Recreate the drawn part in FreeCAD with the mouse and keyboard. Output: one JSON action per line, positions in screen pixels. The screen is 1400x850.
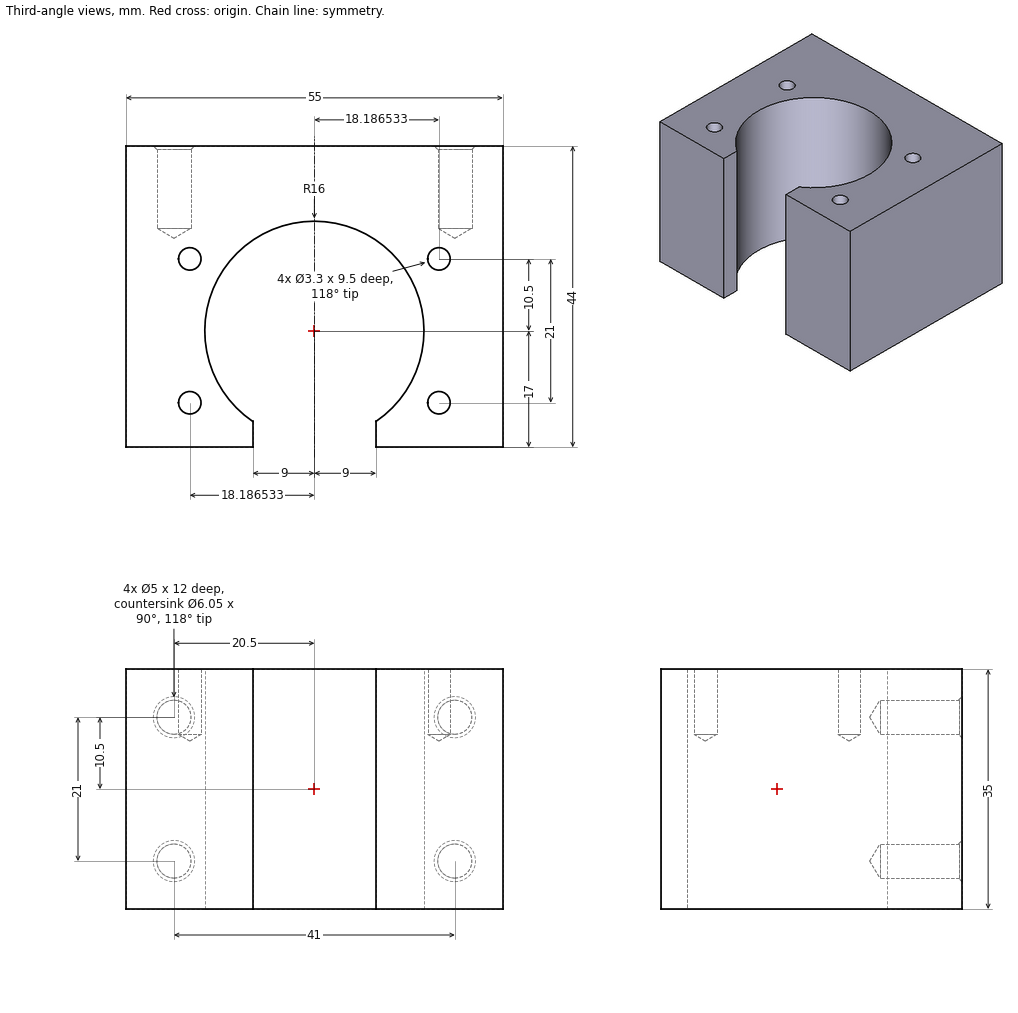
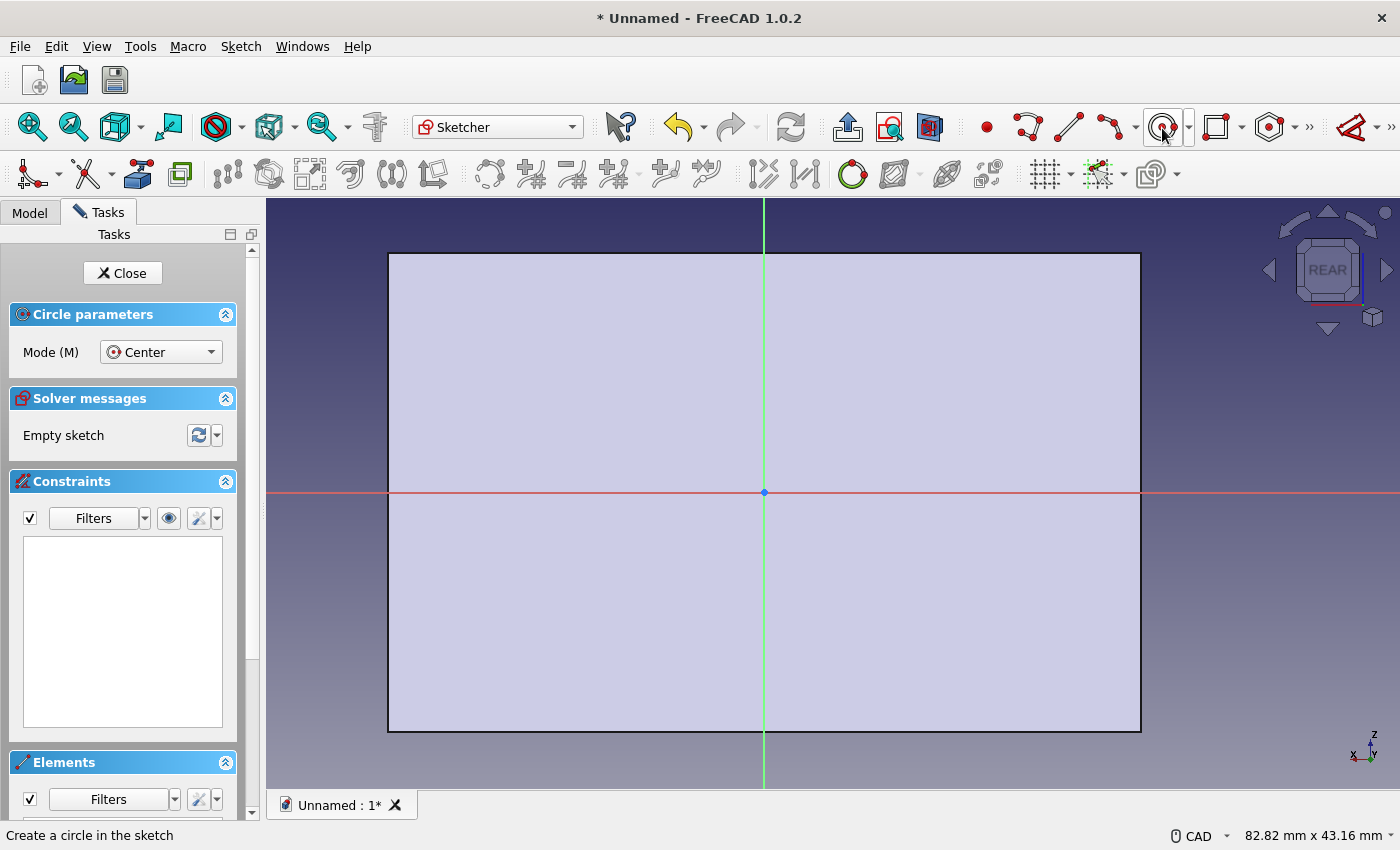
{"action": "left_click", "coordinate": [1045, 349]}
{"action": "mouse_move", "coordinate": [1069, 325]}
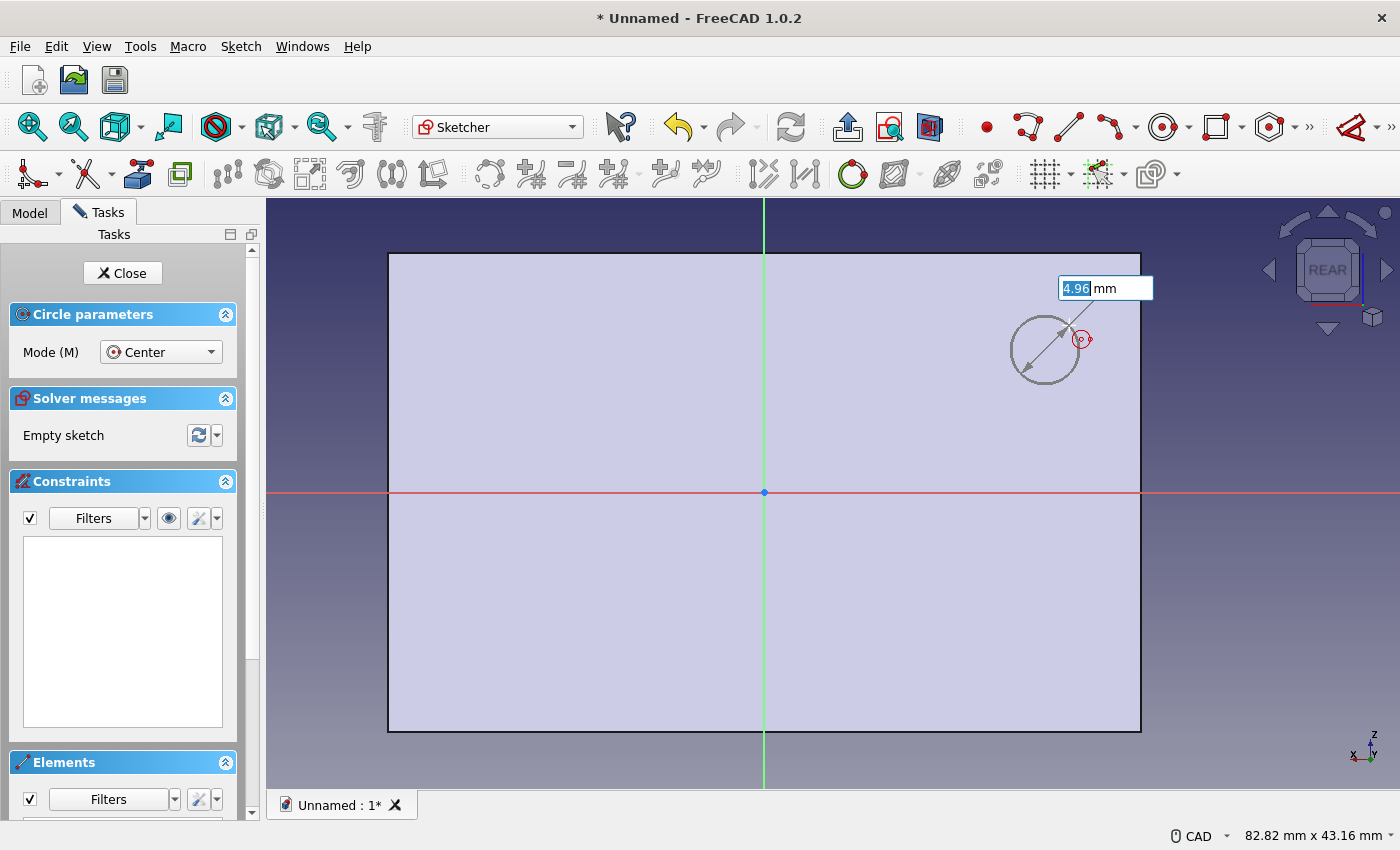
{"action": "type", "text": "5"}
{"action": "key", "text": "Return"}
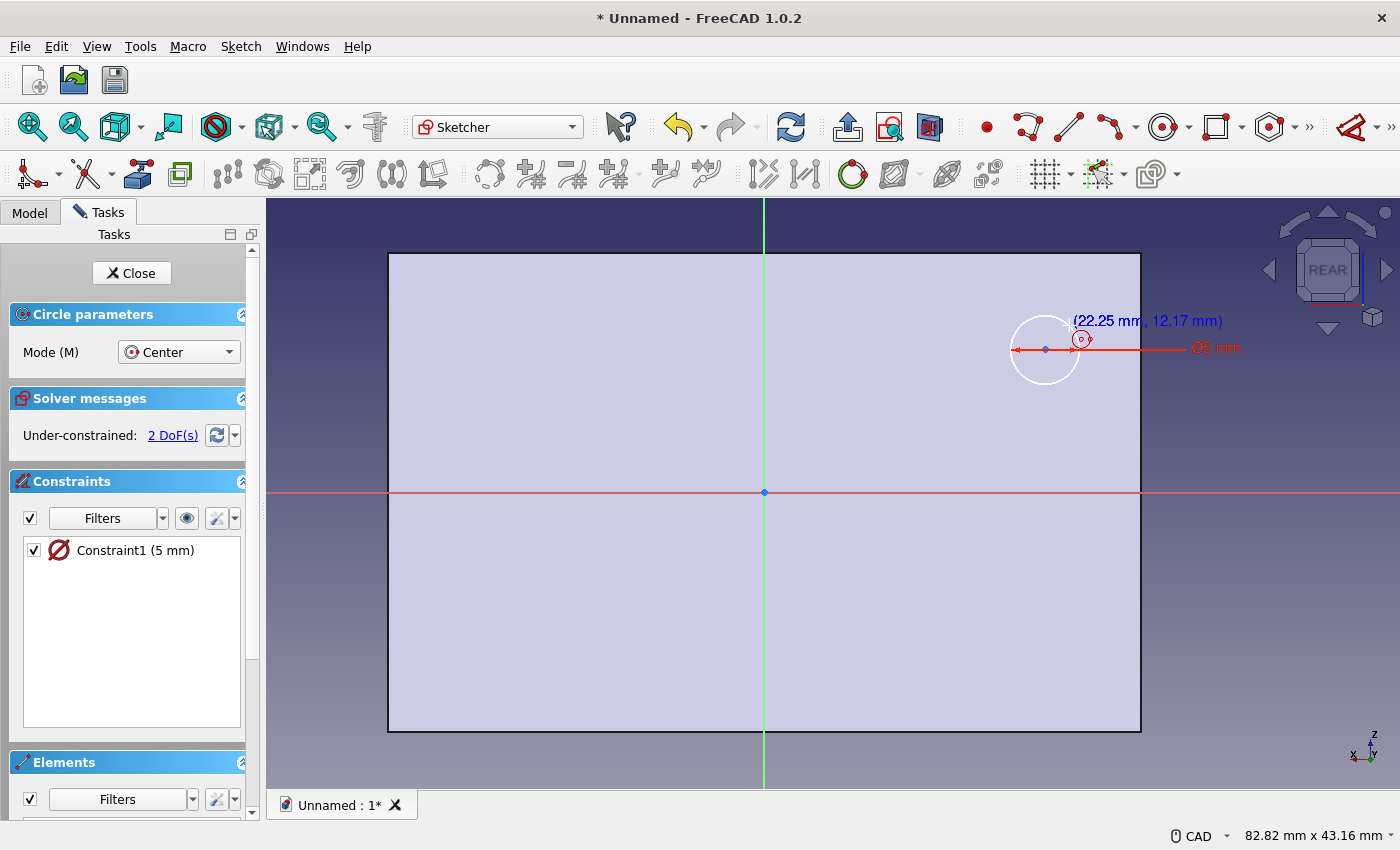
{"action": "left_click", "coordinate": [1045, 636]}
{"action": "mouse_move", "coordinate": [1069, 612]}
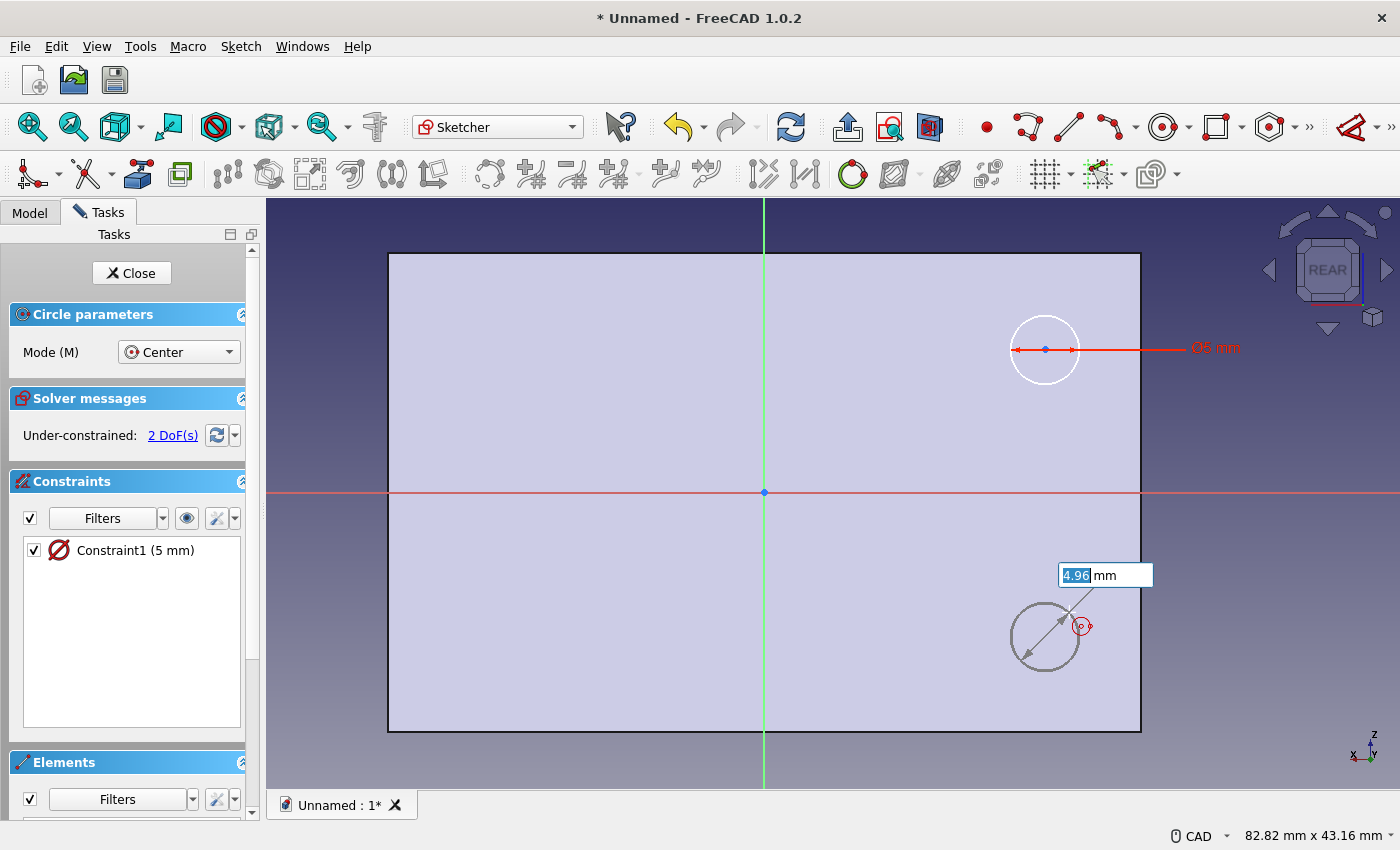
{"action": "type", "text": "5"}
{"action": "key", "text": "Return"}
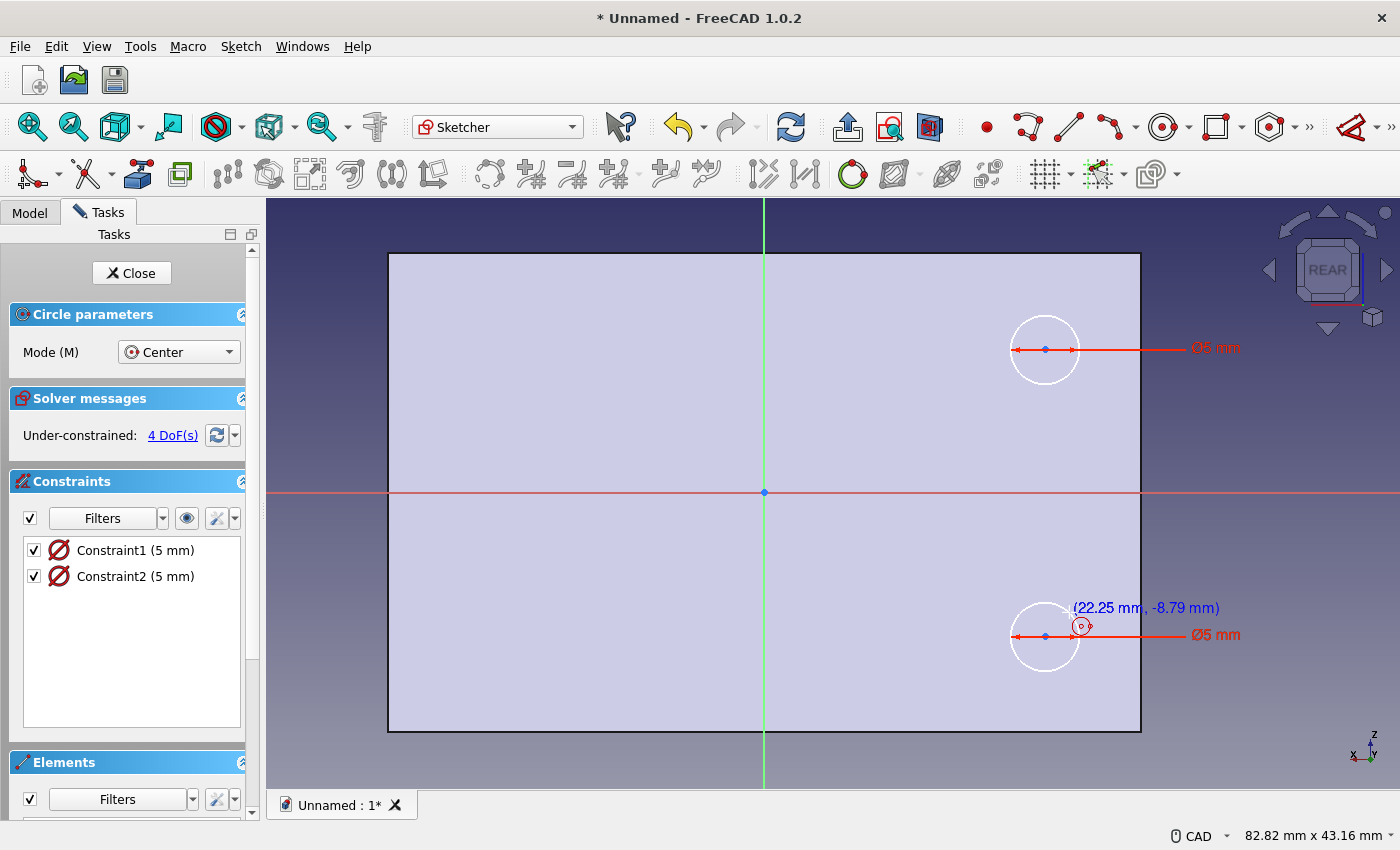
{"action": "left_click", "coordinate": [484, 636]}
{"action": "mouse_move", "coordinate": [508, 612]}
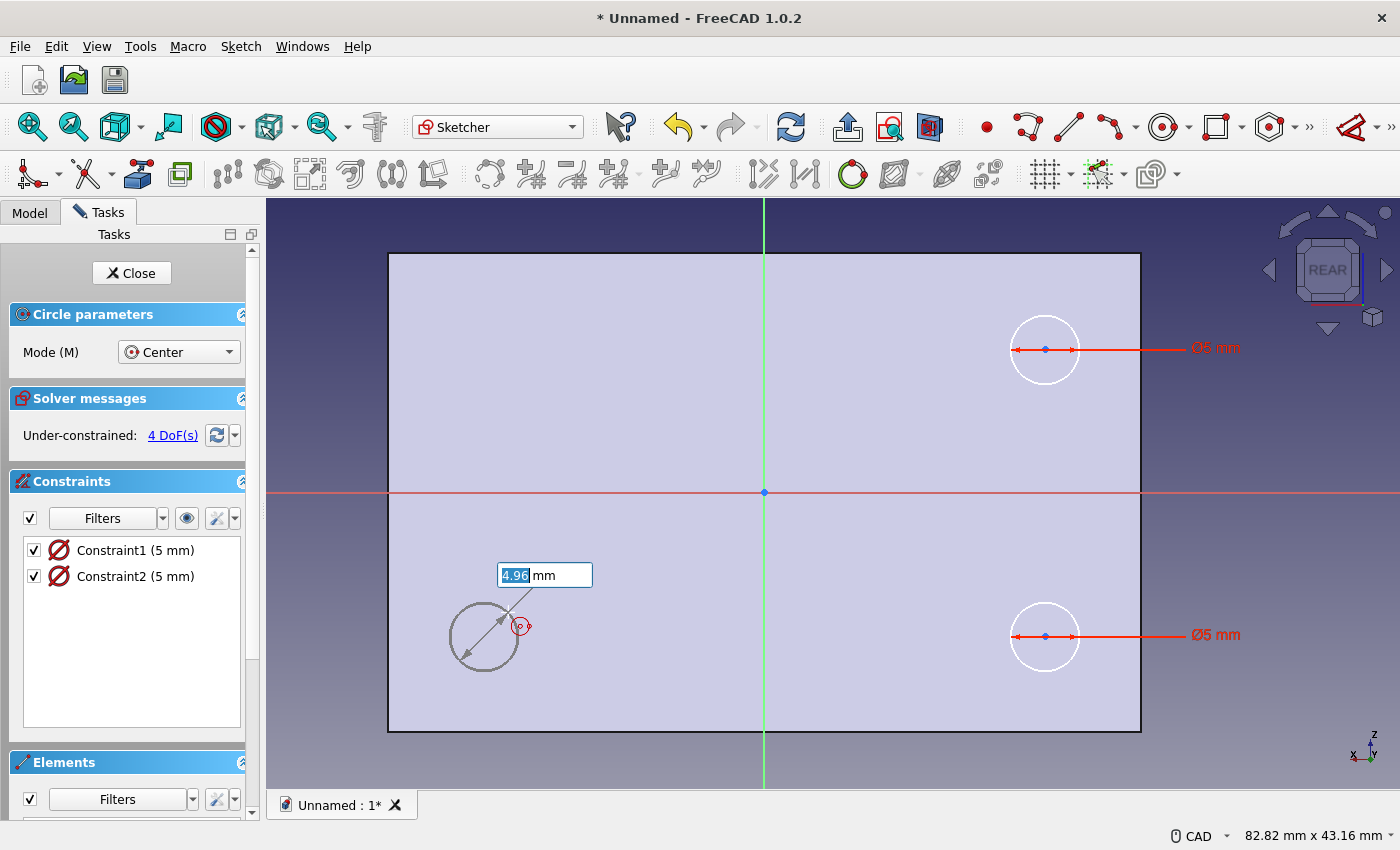
{"action": "type", "text": "5"}
{"action": "key", "text": "Return"}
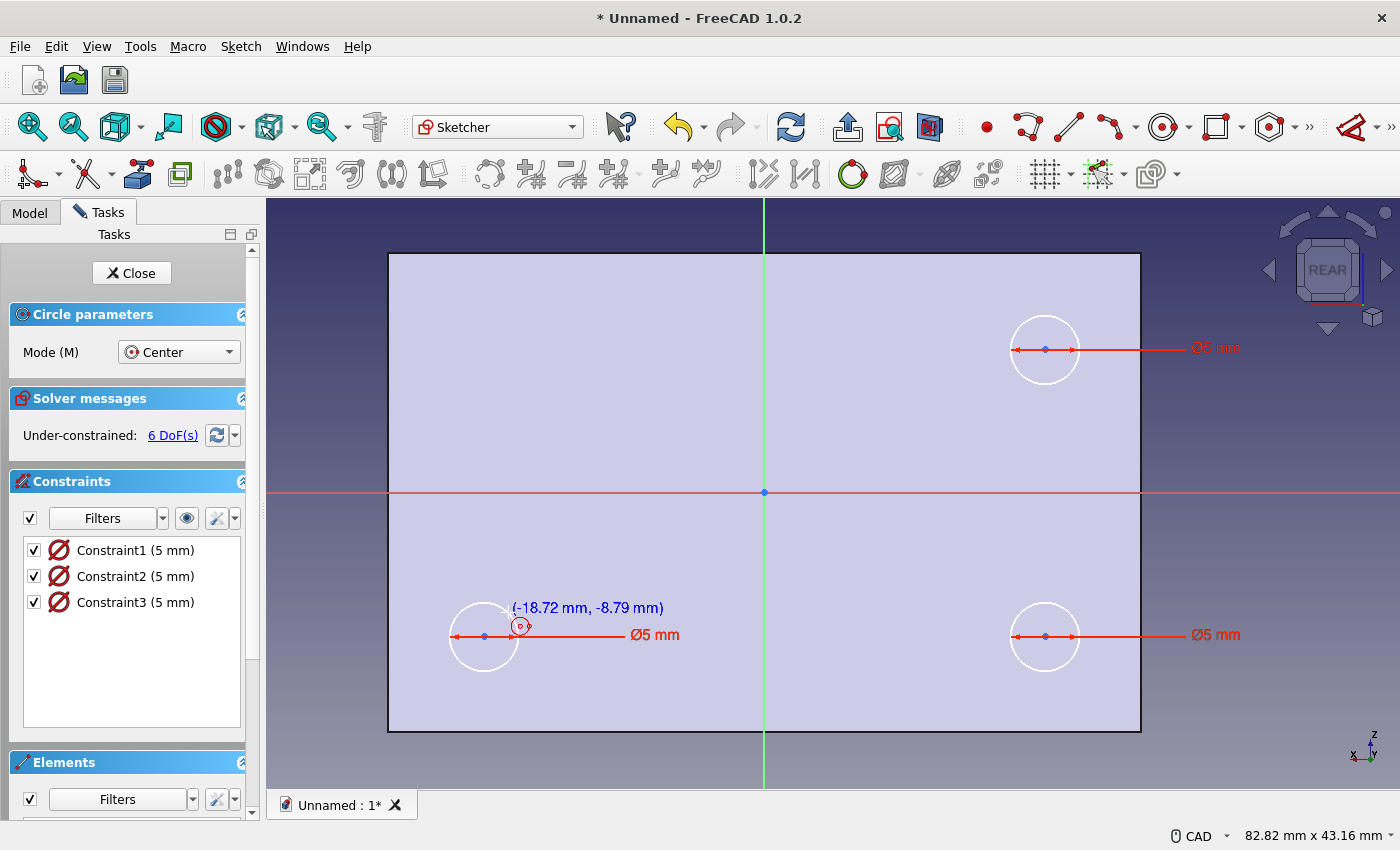
{"action": "left_click", "coordinate": [484, 349]}
{"action": "mouse_move", "coordinate": [508, 325]}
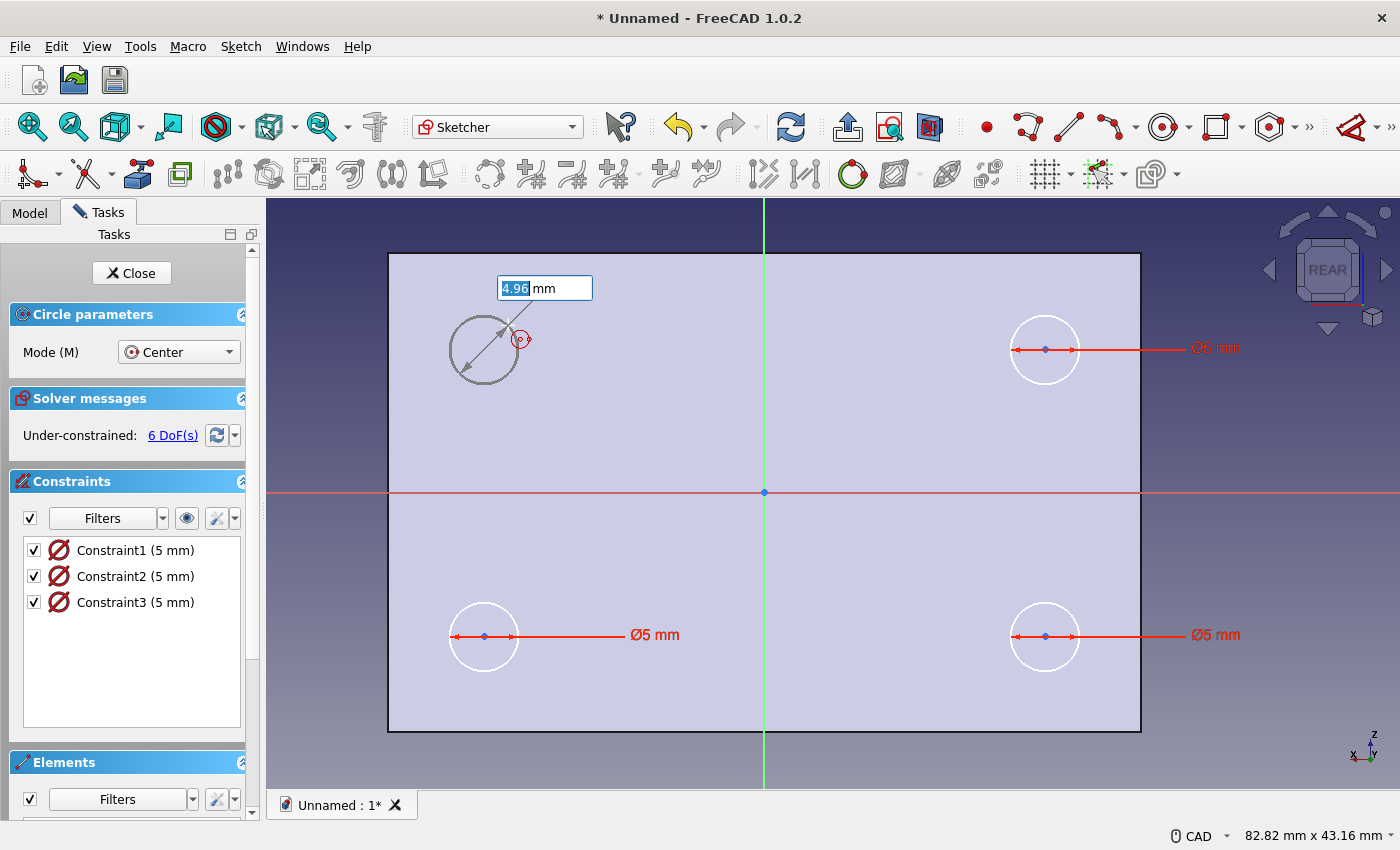
{"action": "type", "text": "5"}
{"action": "key", "text": "Return"}
{"action": "key", "text": "Escape"}